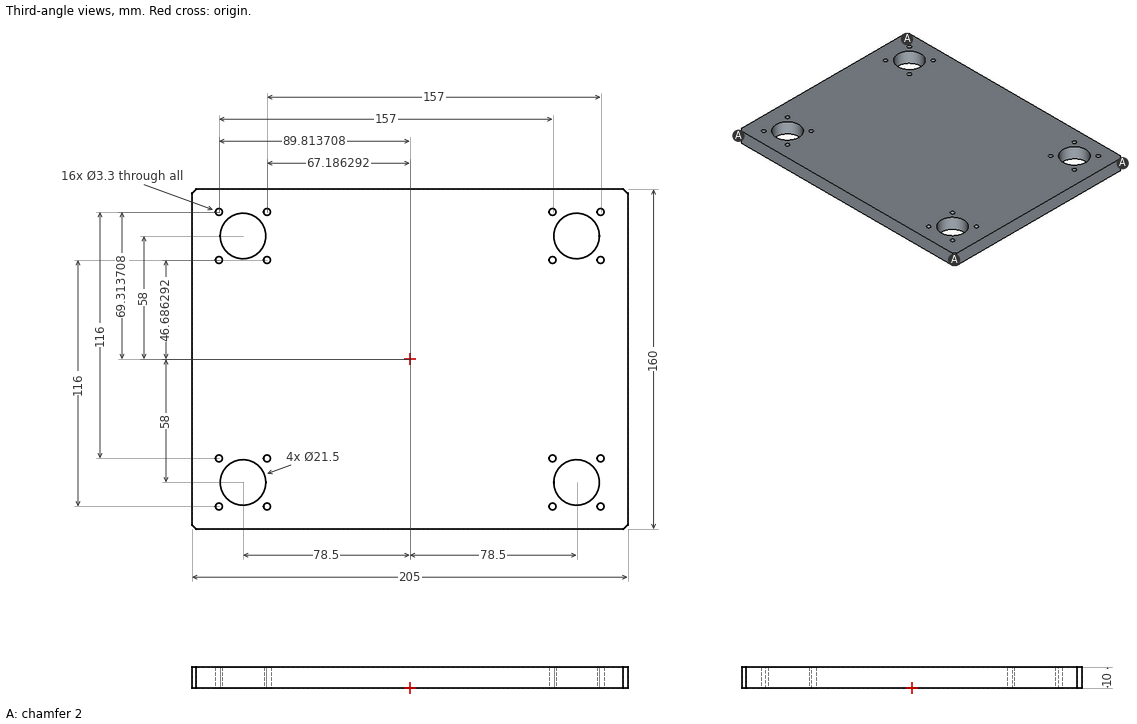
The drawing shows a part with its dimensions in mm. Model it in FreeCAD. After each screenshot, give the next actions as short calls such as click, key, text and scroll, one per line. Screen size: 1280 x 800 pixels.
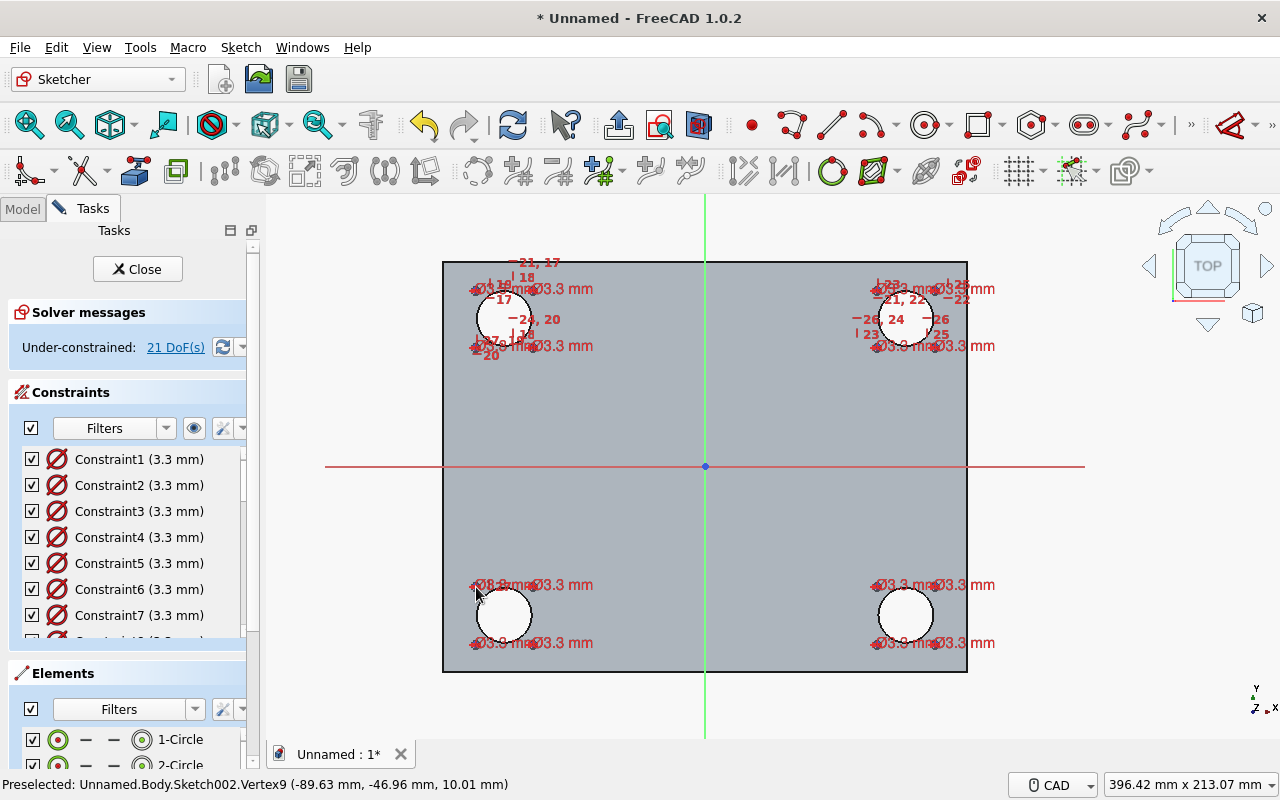
click(533, 348)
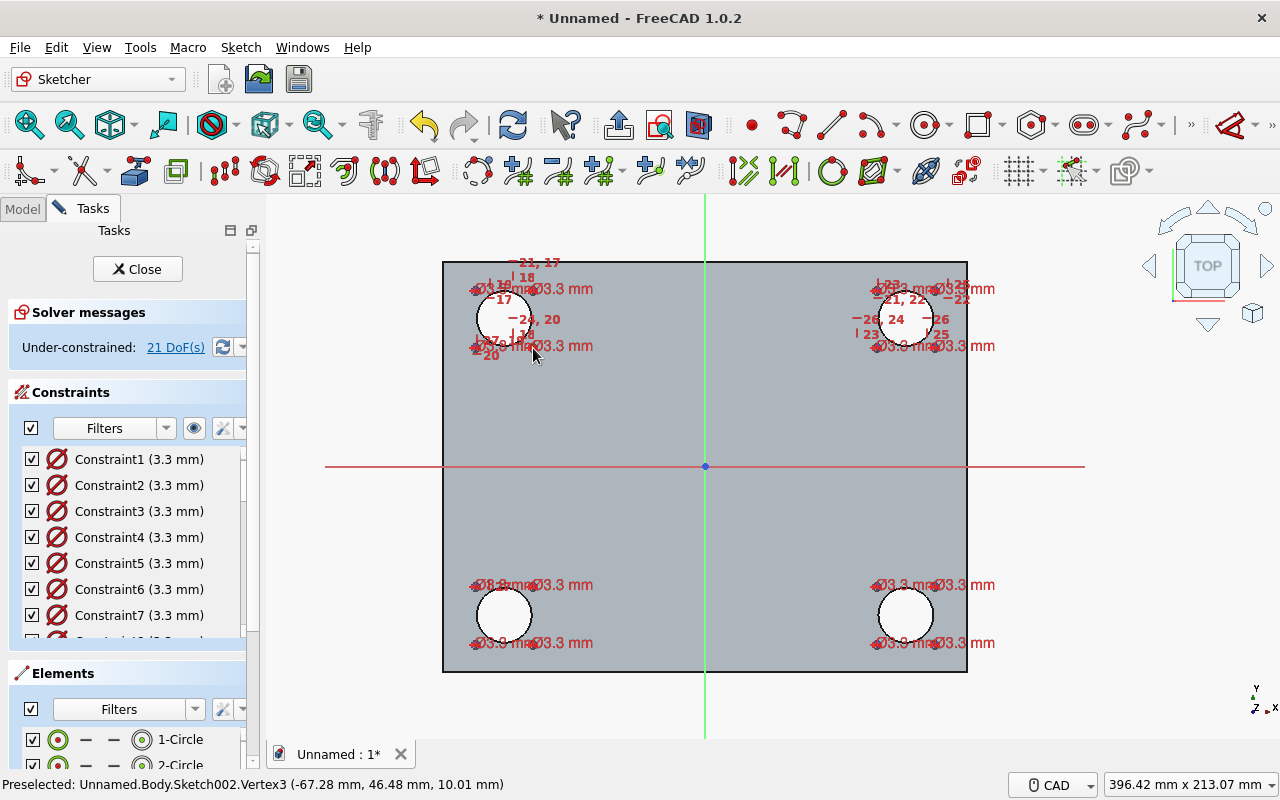
click(533, 587)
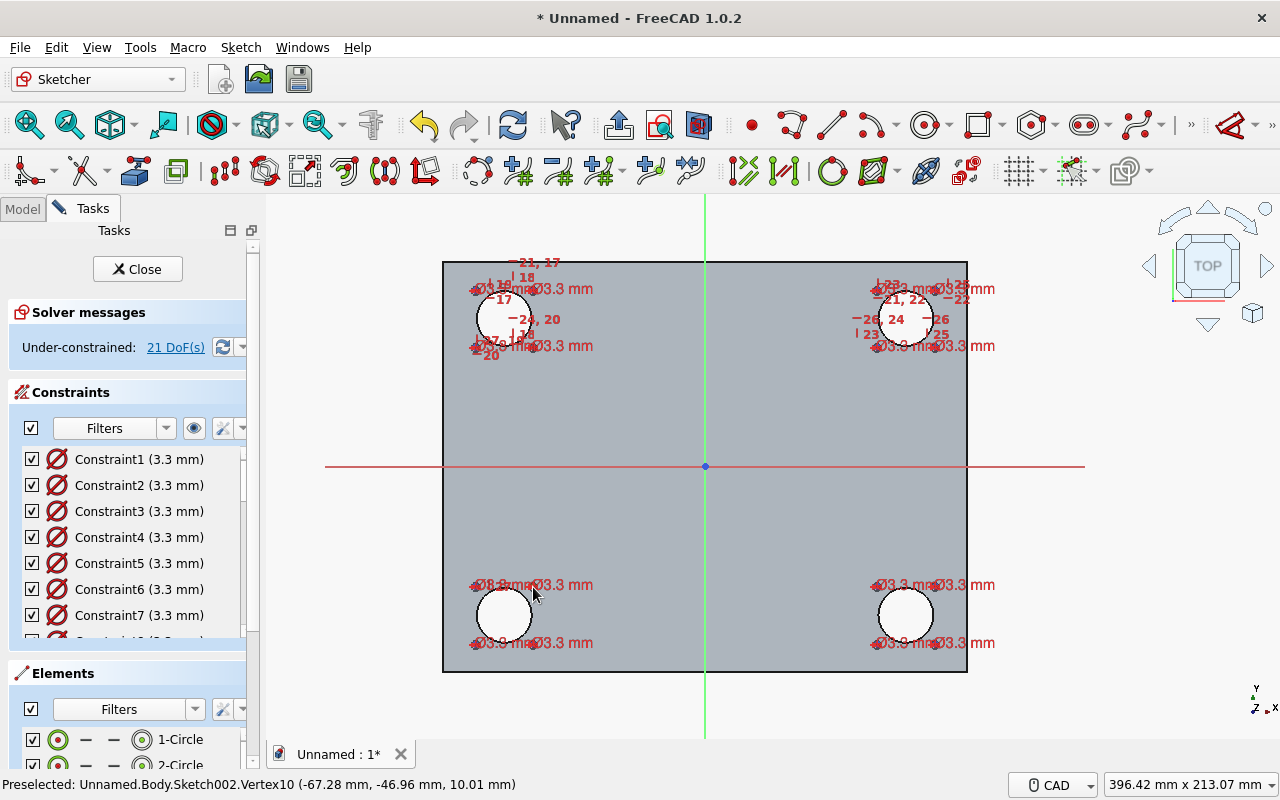
key(v)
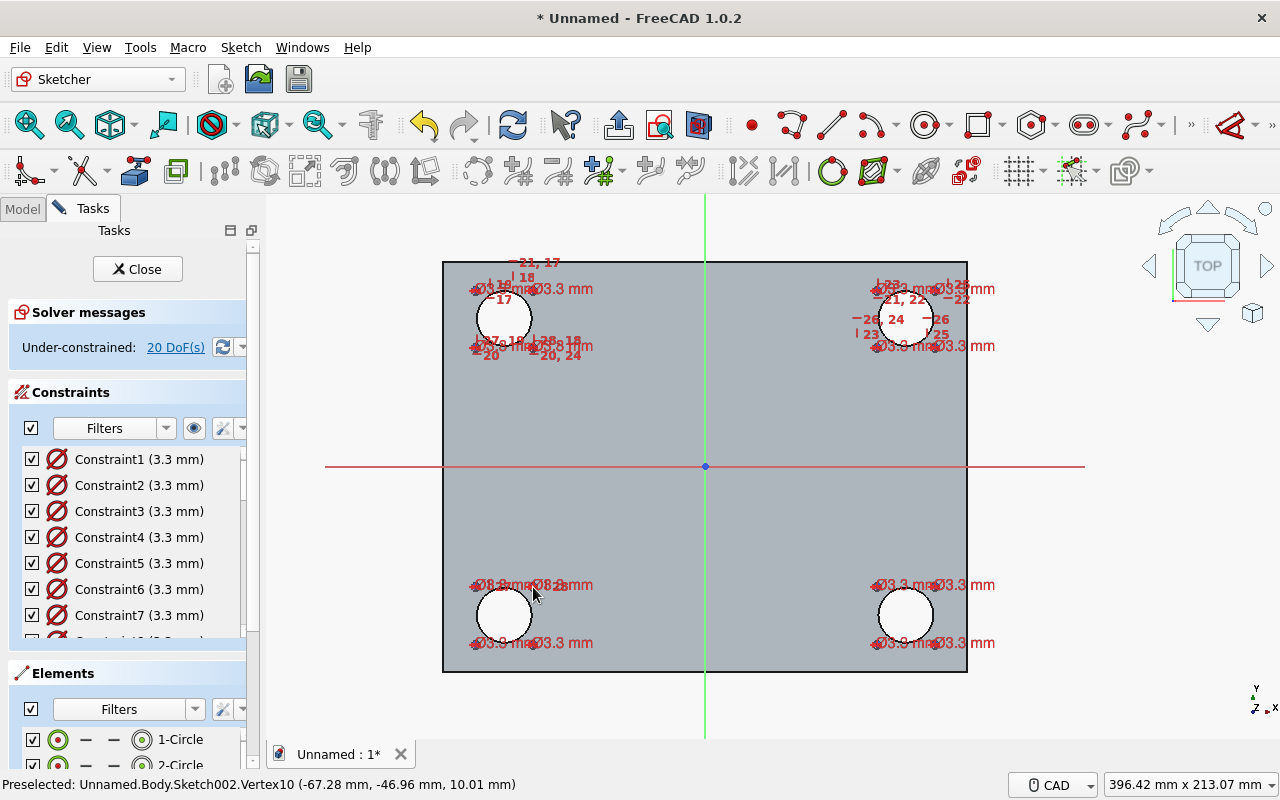
click(476, 587)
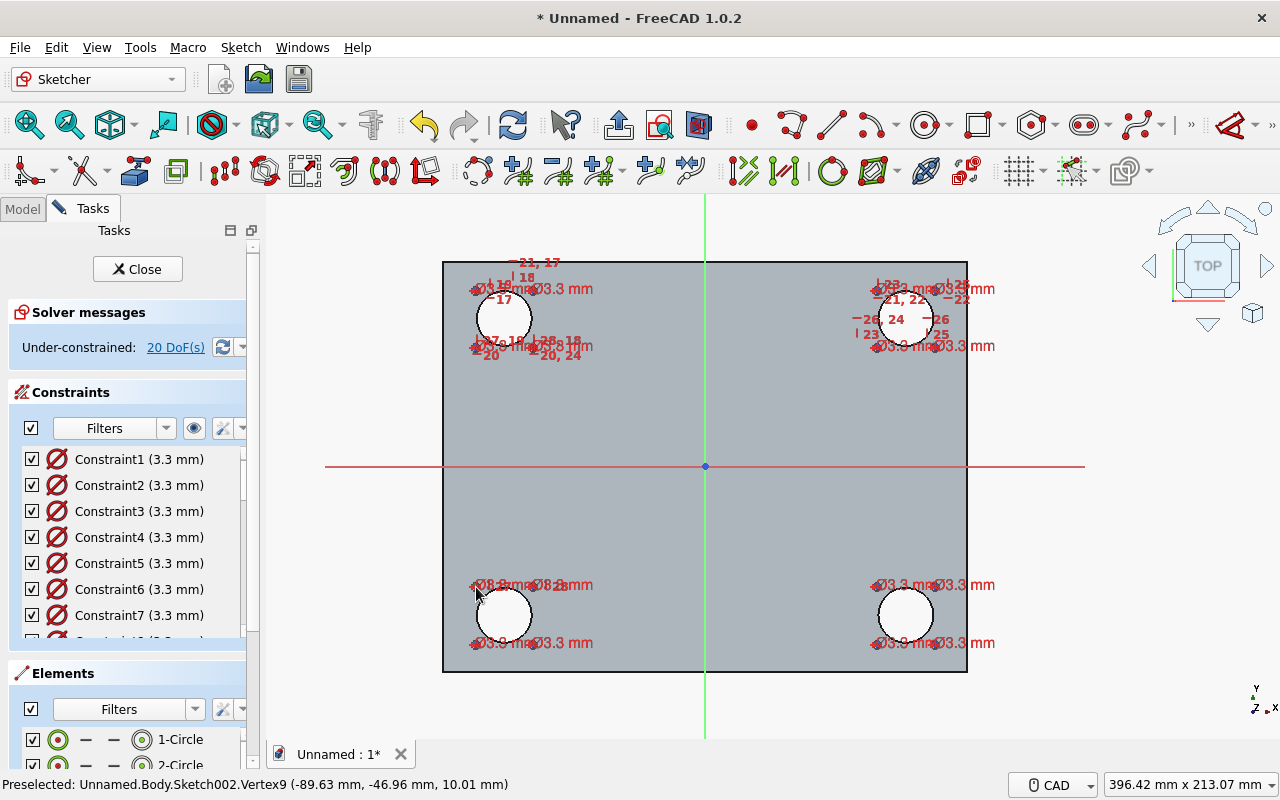
click(533, 587)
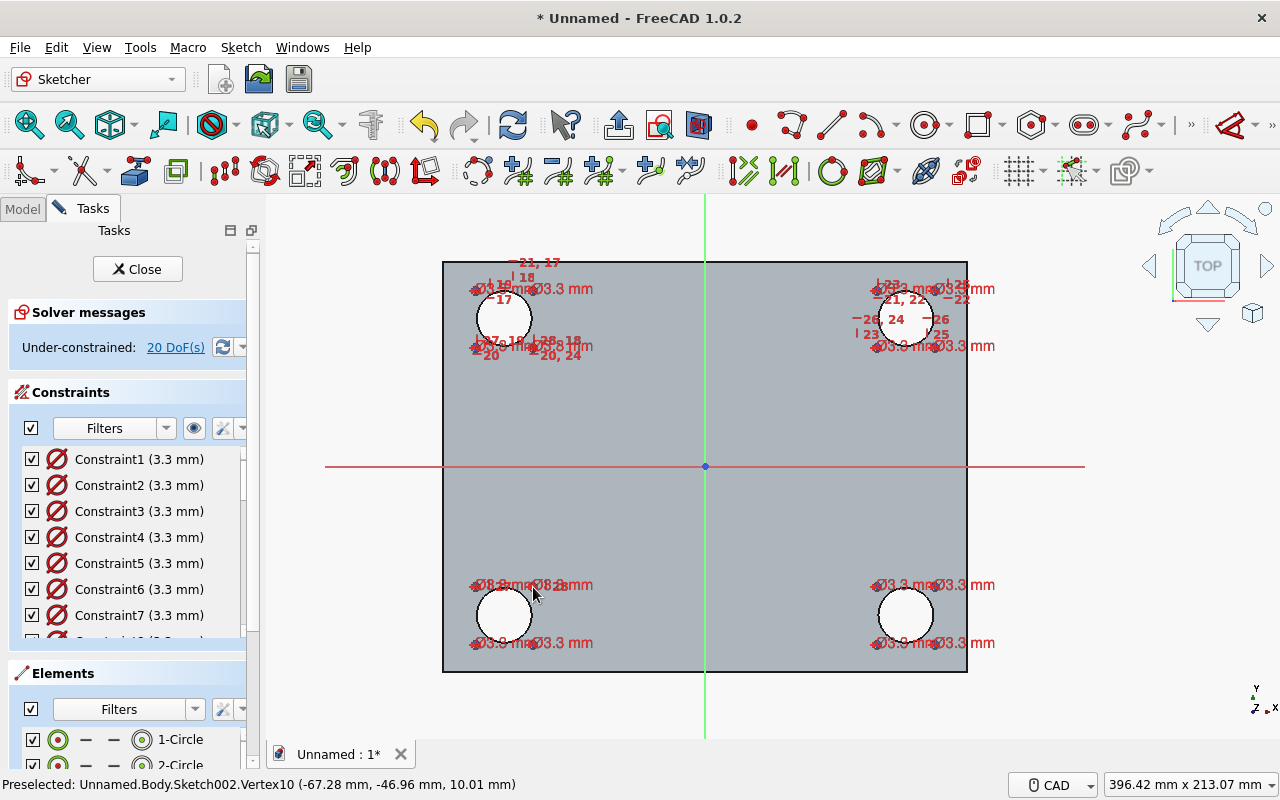
key(h)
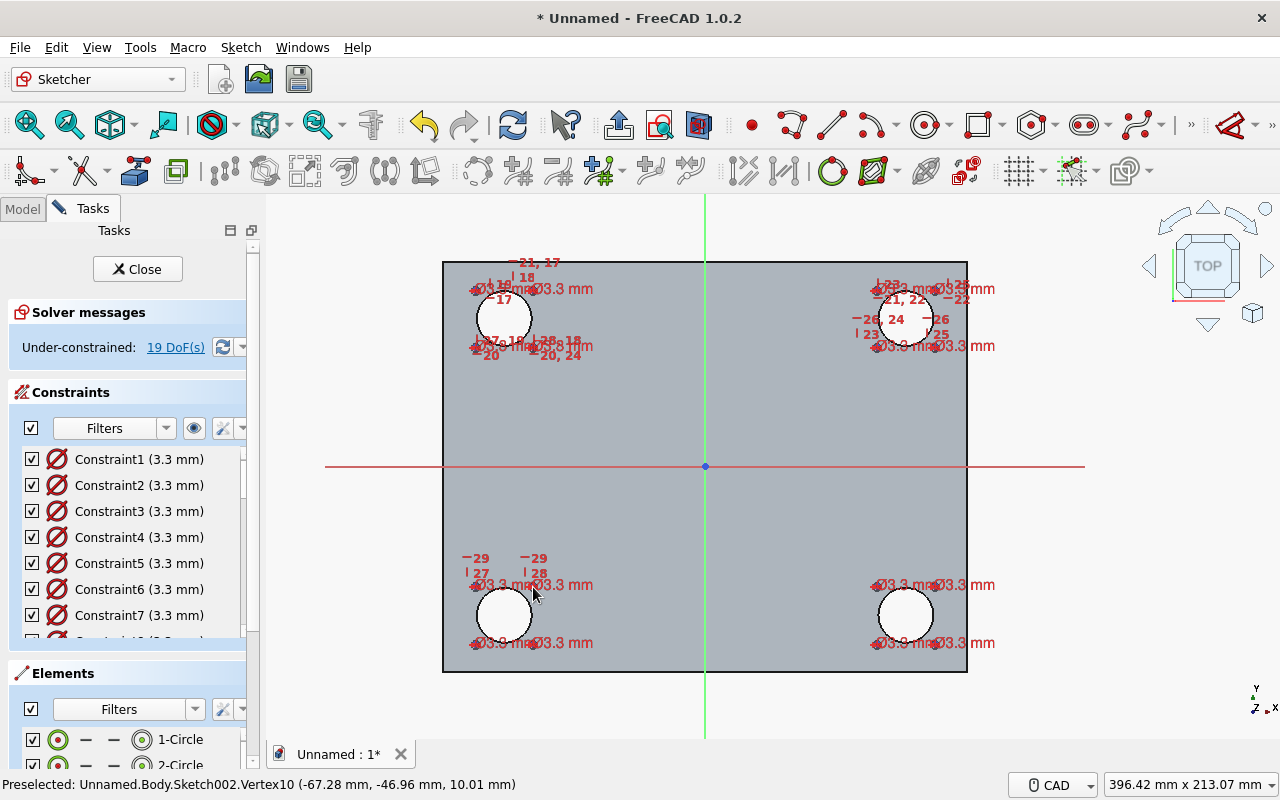
click(476, 587)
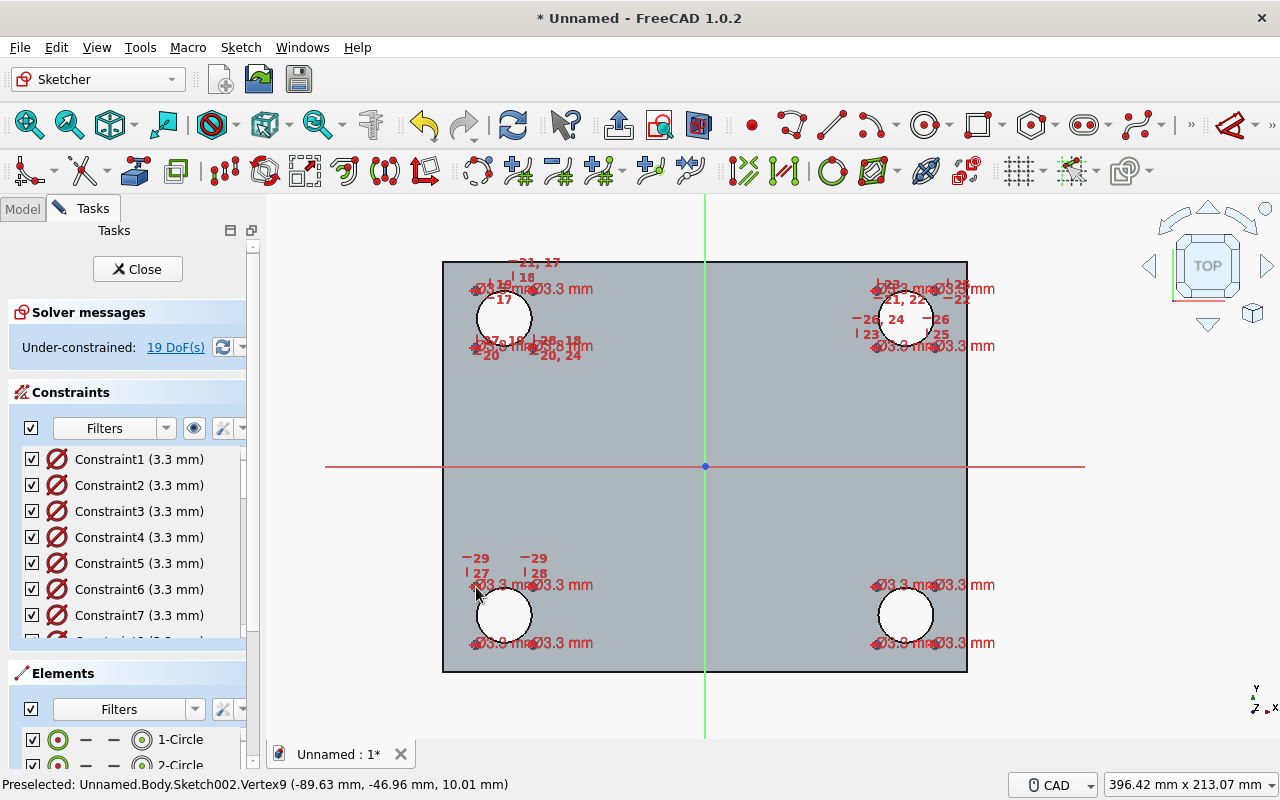
click(476, 645)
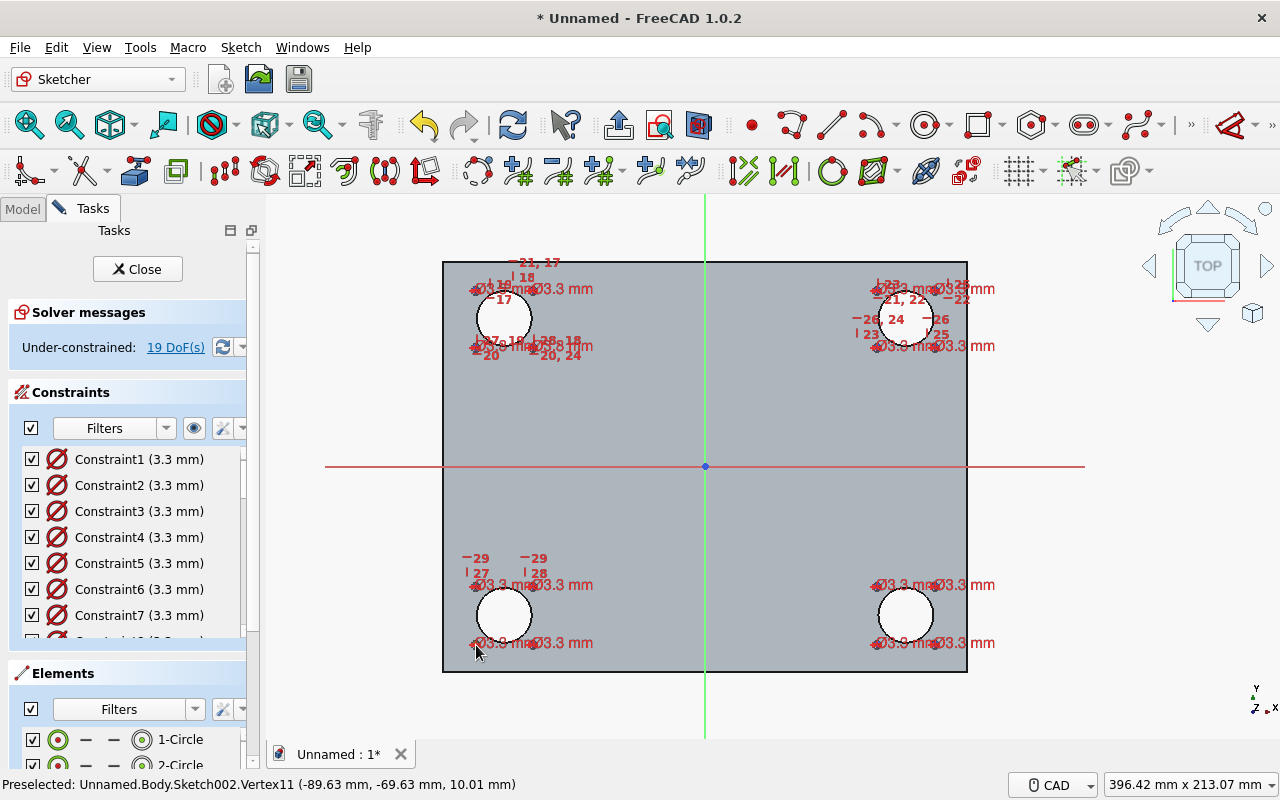
key(v)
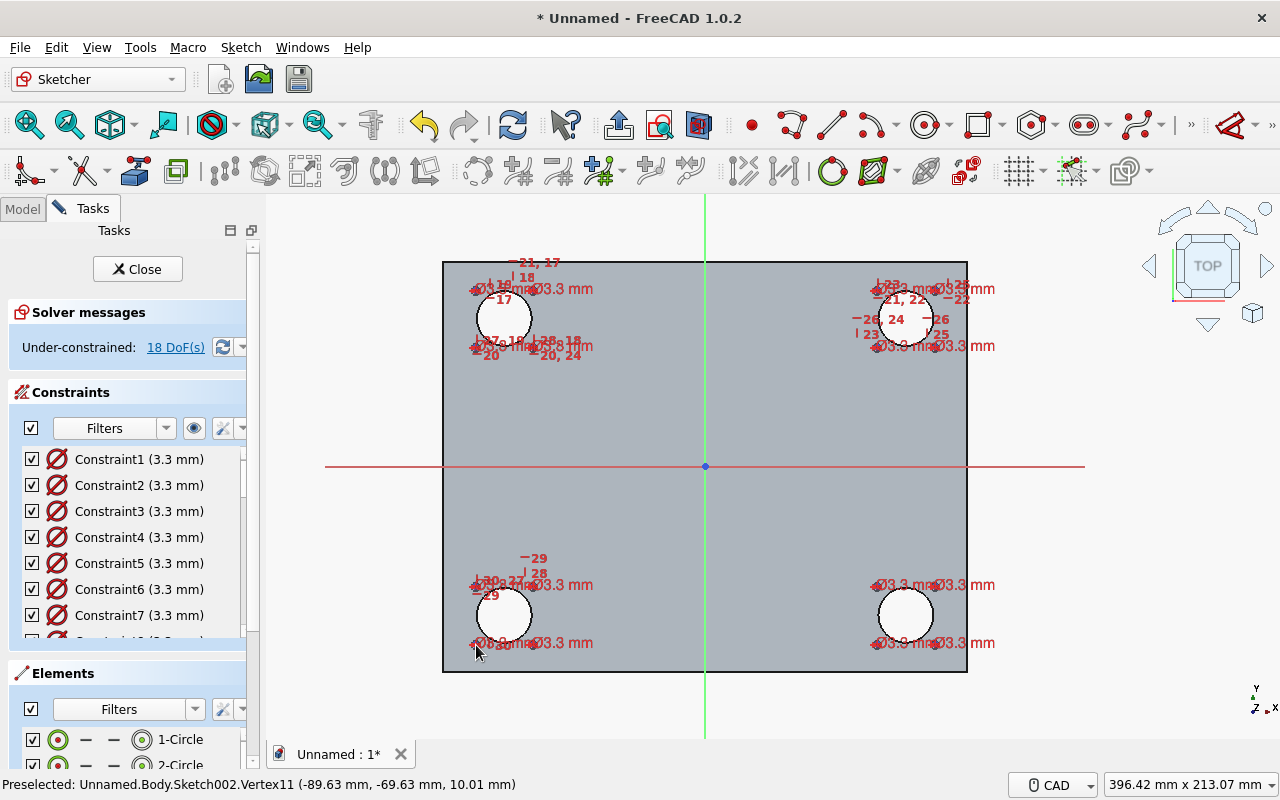
click(533, 587)